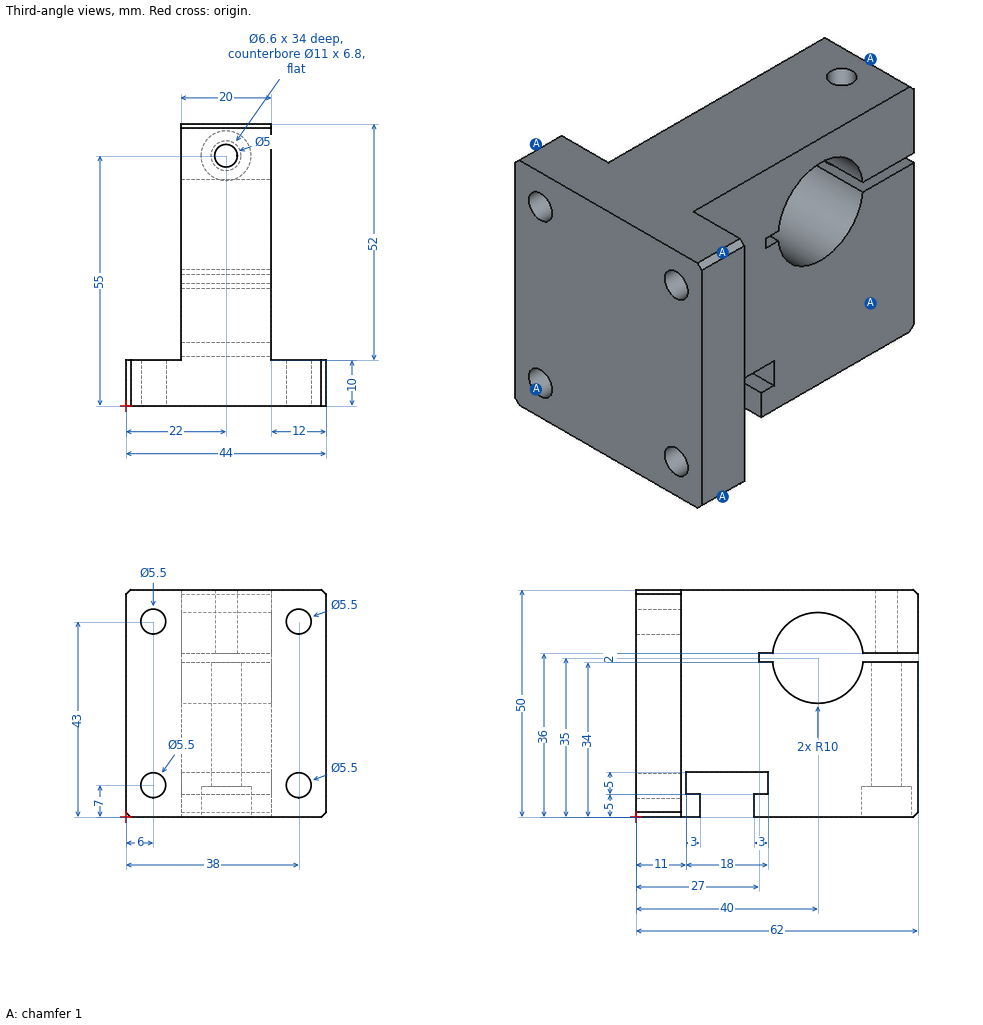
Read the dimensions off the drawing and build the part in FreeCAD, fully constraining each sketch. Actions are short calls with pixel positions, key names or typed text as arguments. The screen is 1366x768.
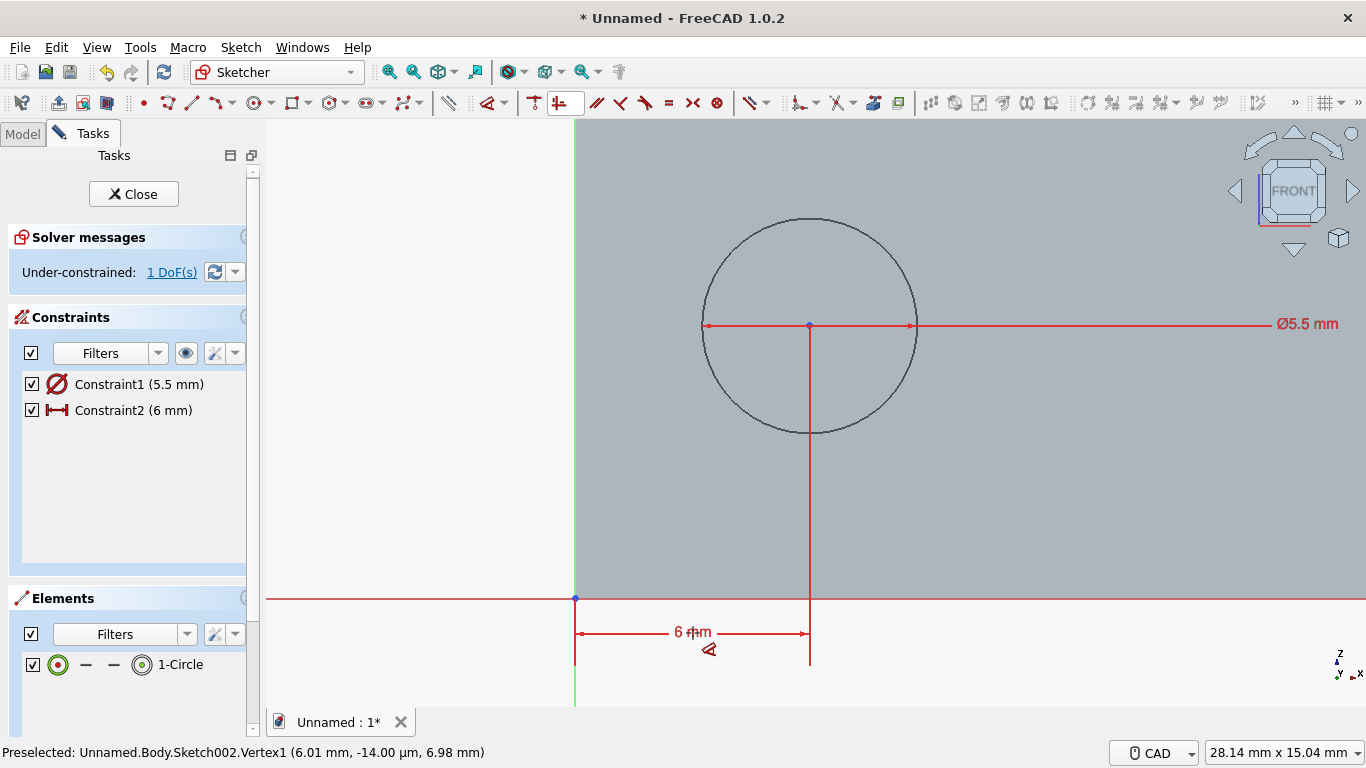
click(810, 326)
click(541, 462)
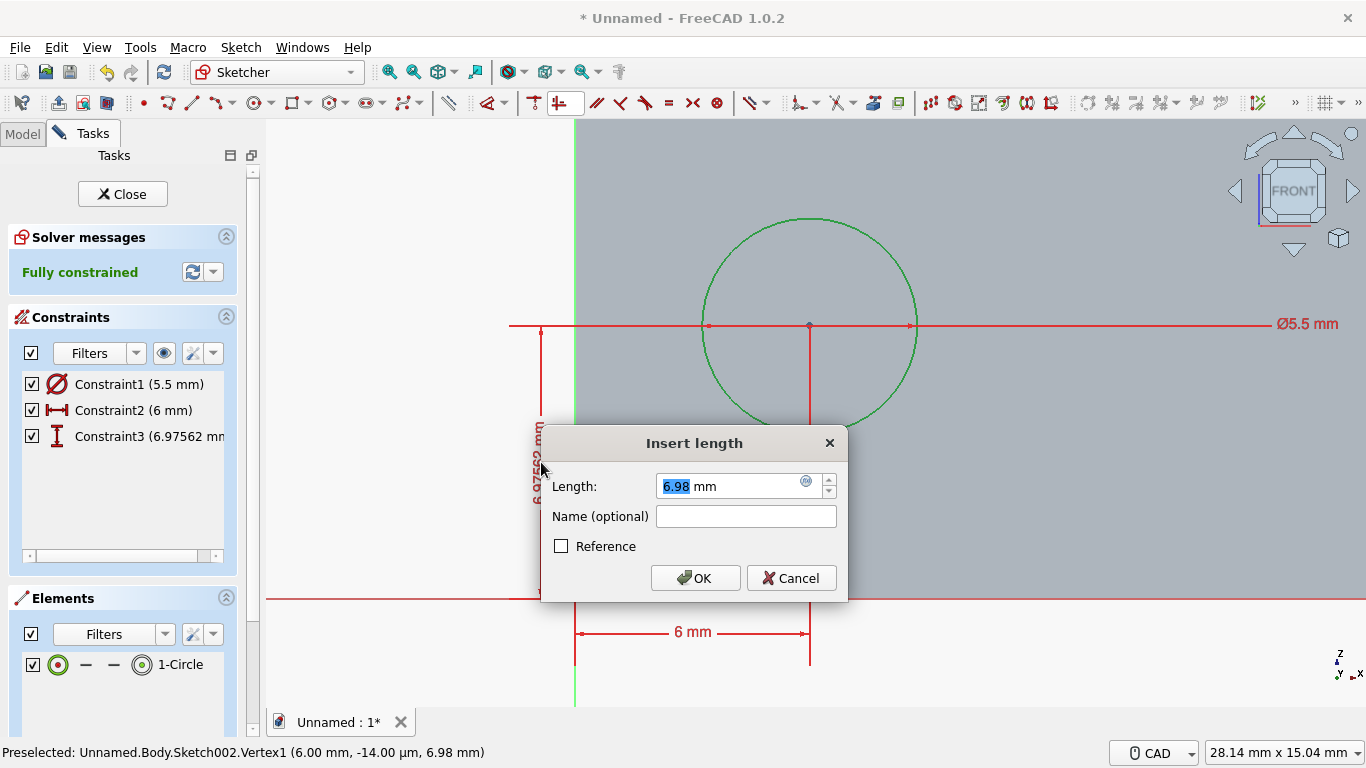
text(7)
key(Return)
key(Escape)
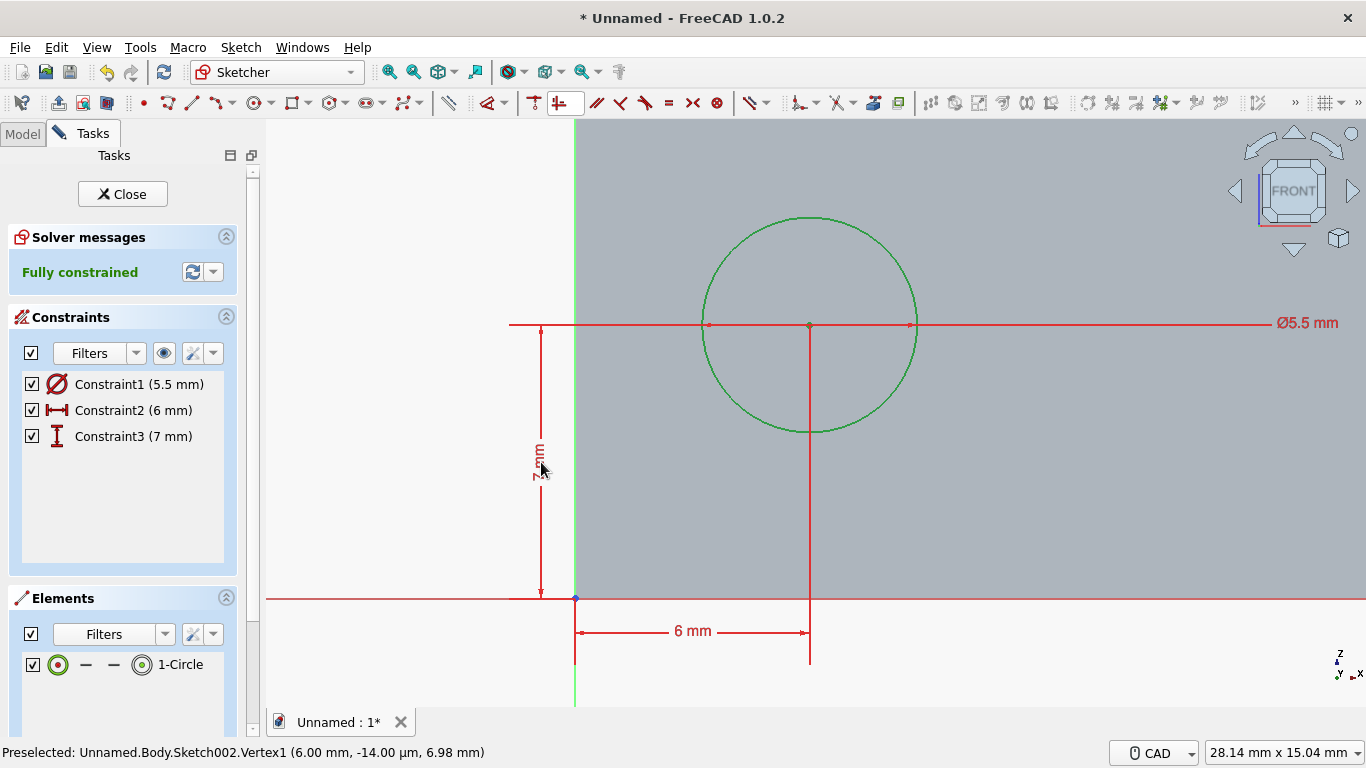
click(123, 194)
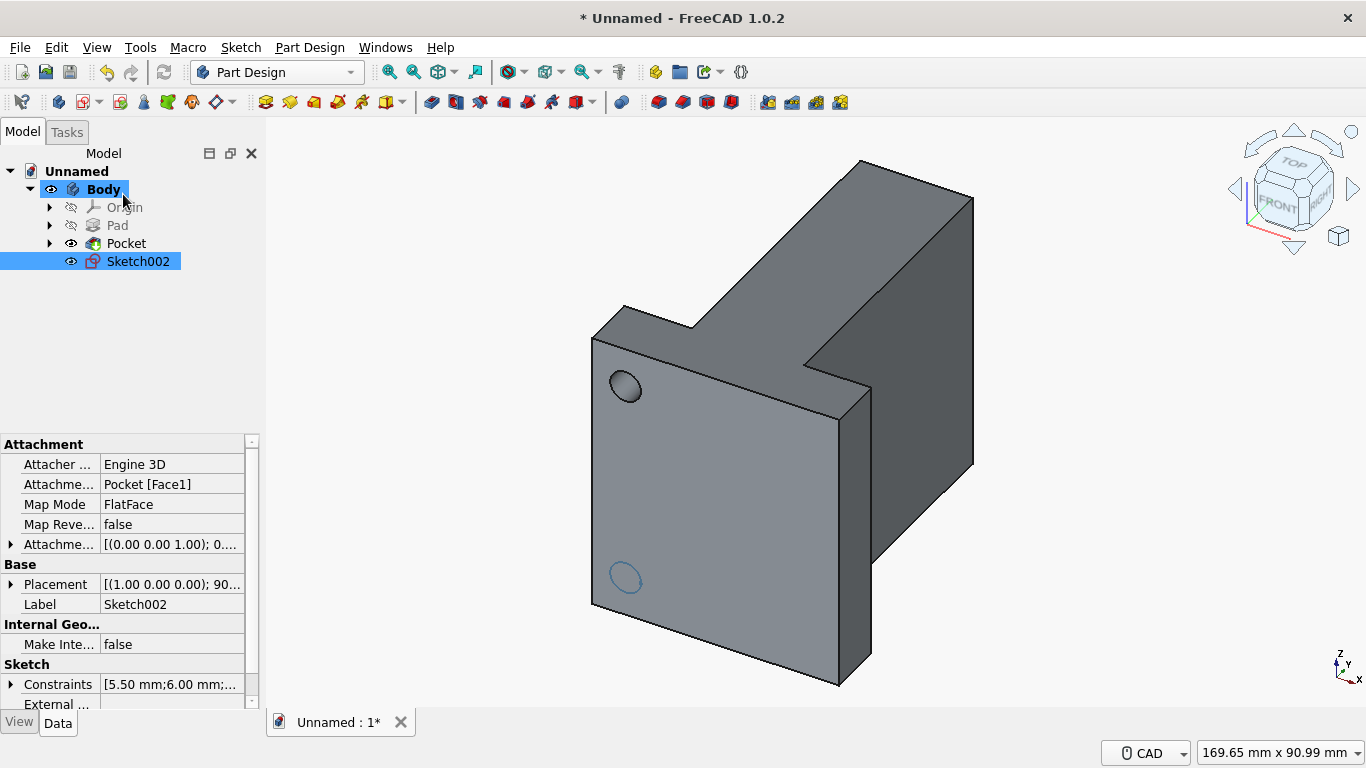
click(432, 102)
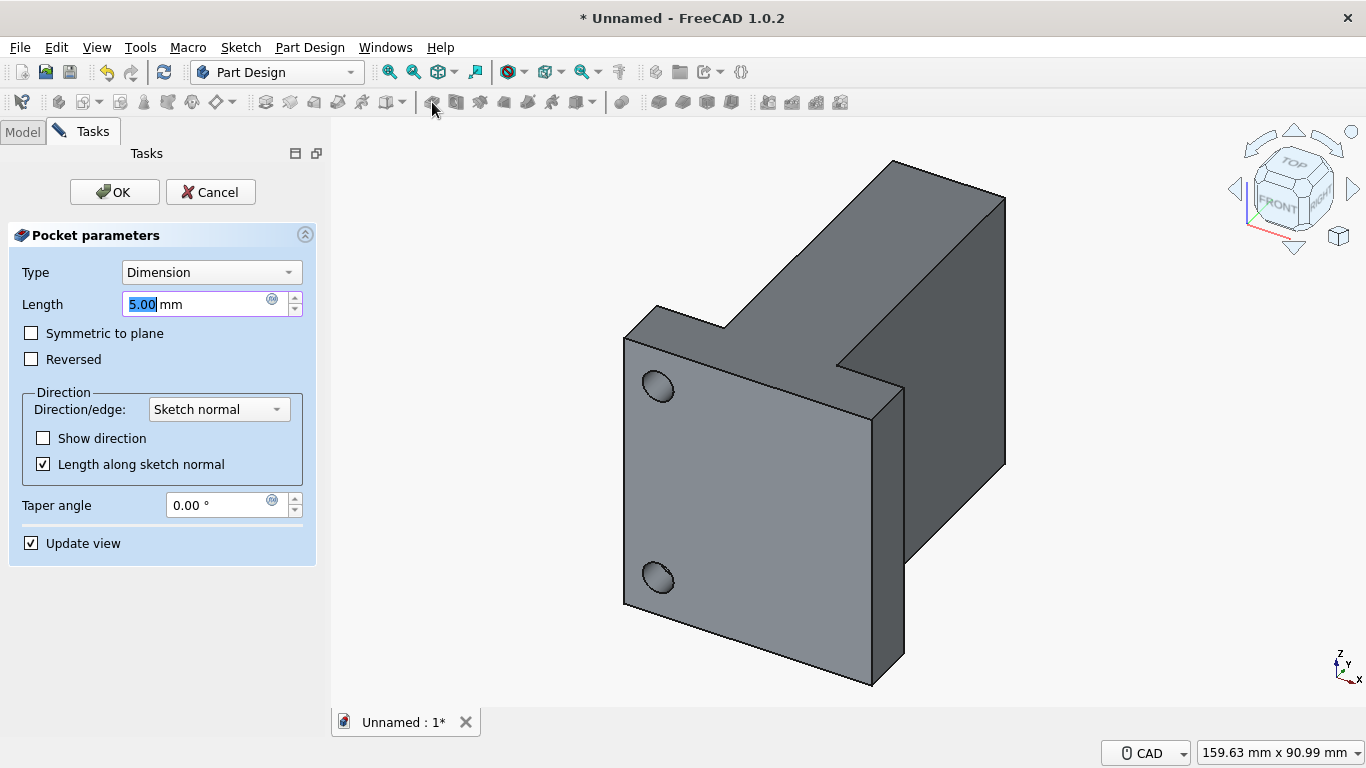
click(212, 272)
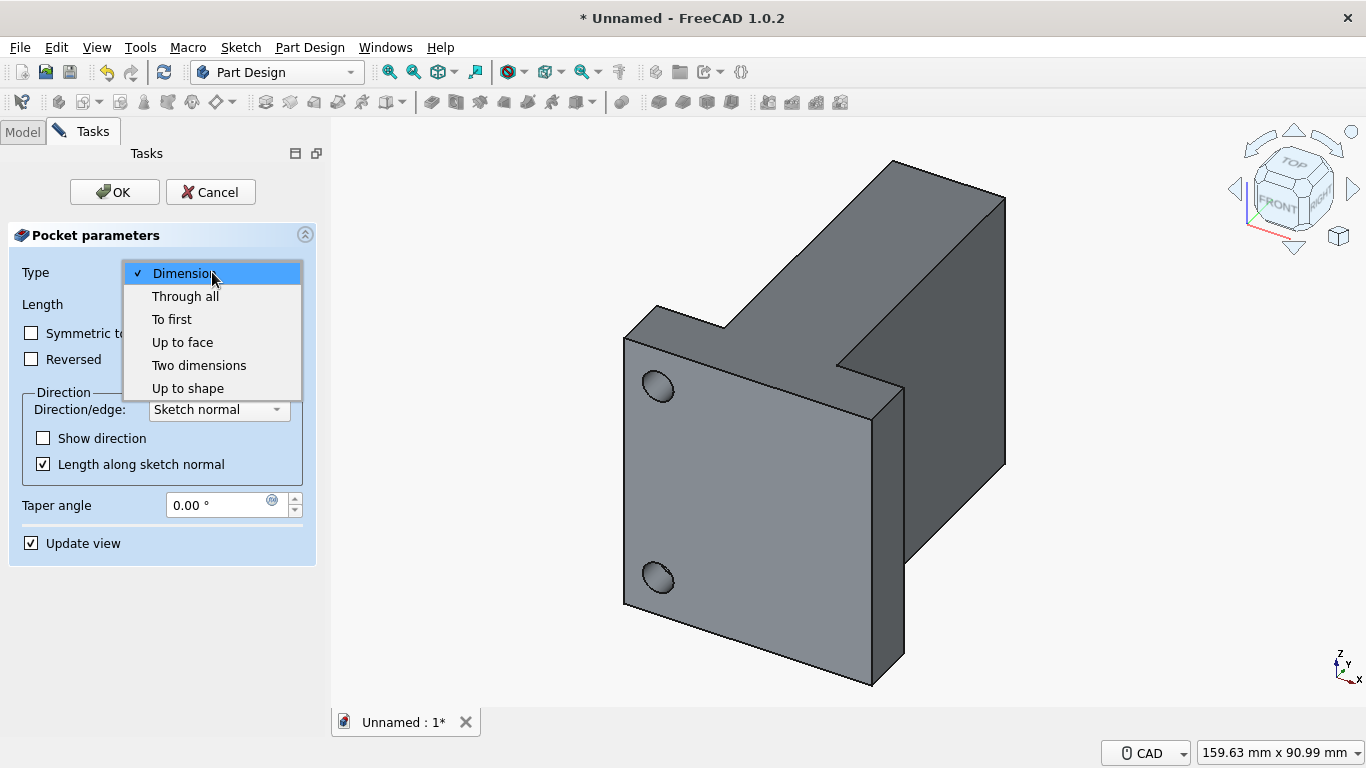
click(212, 320)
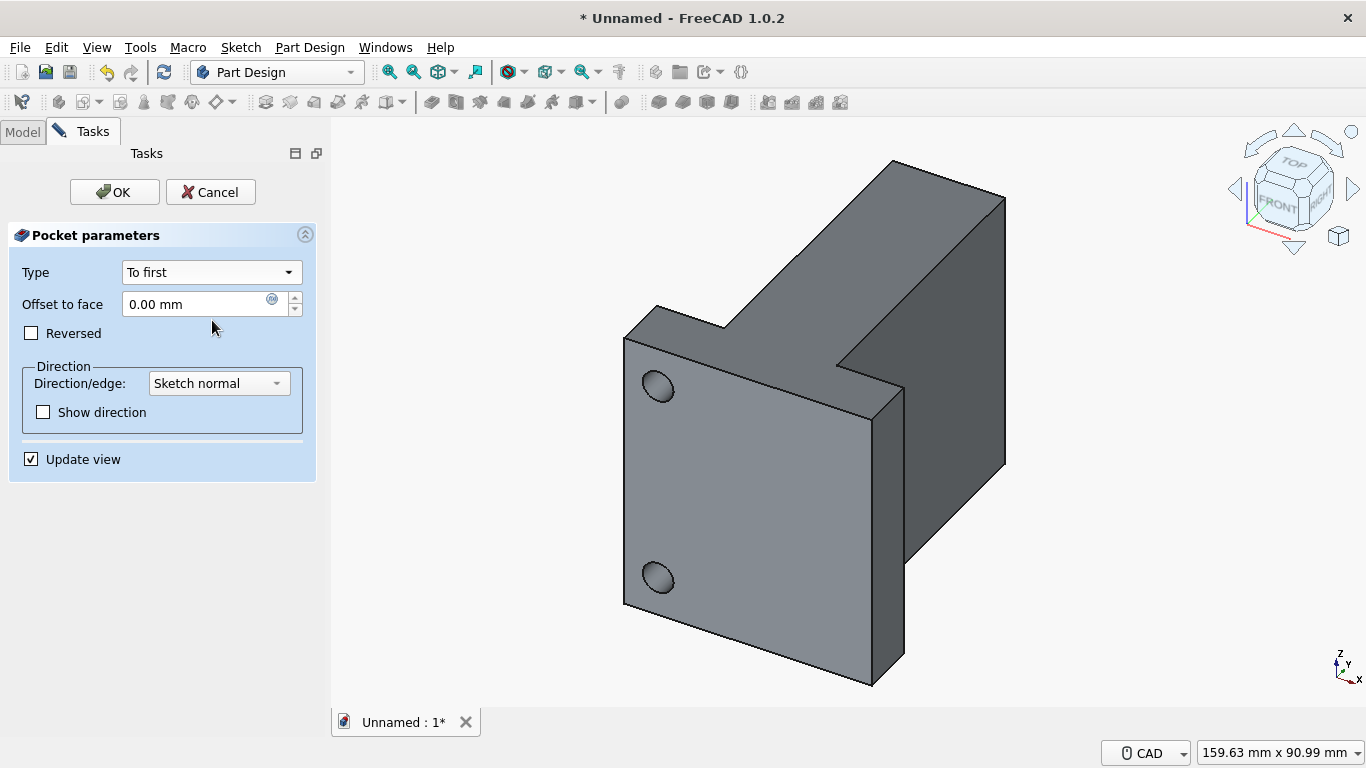
click(115, 192)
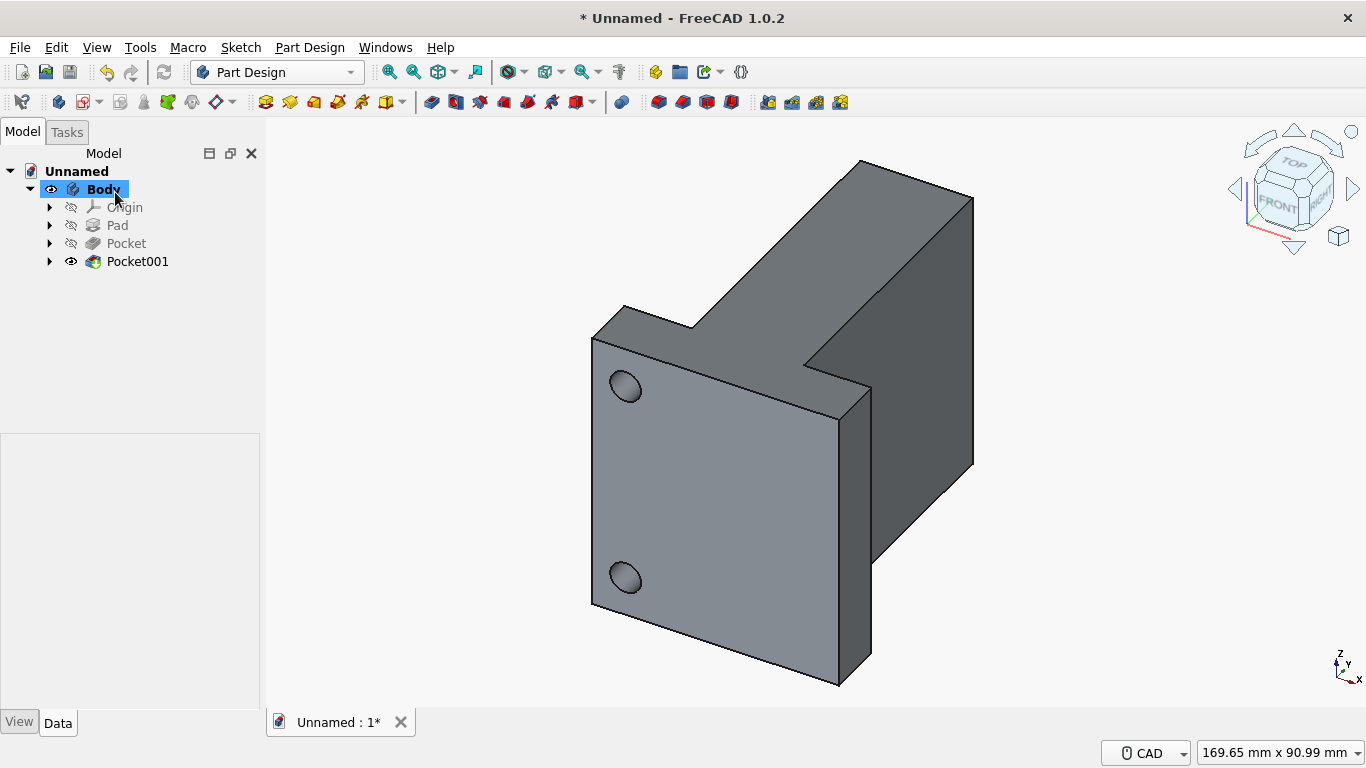
click(715, 511)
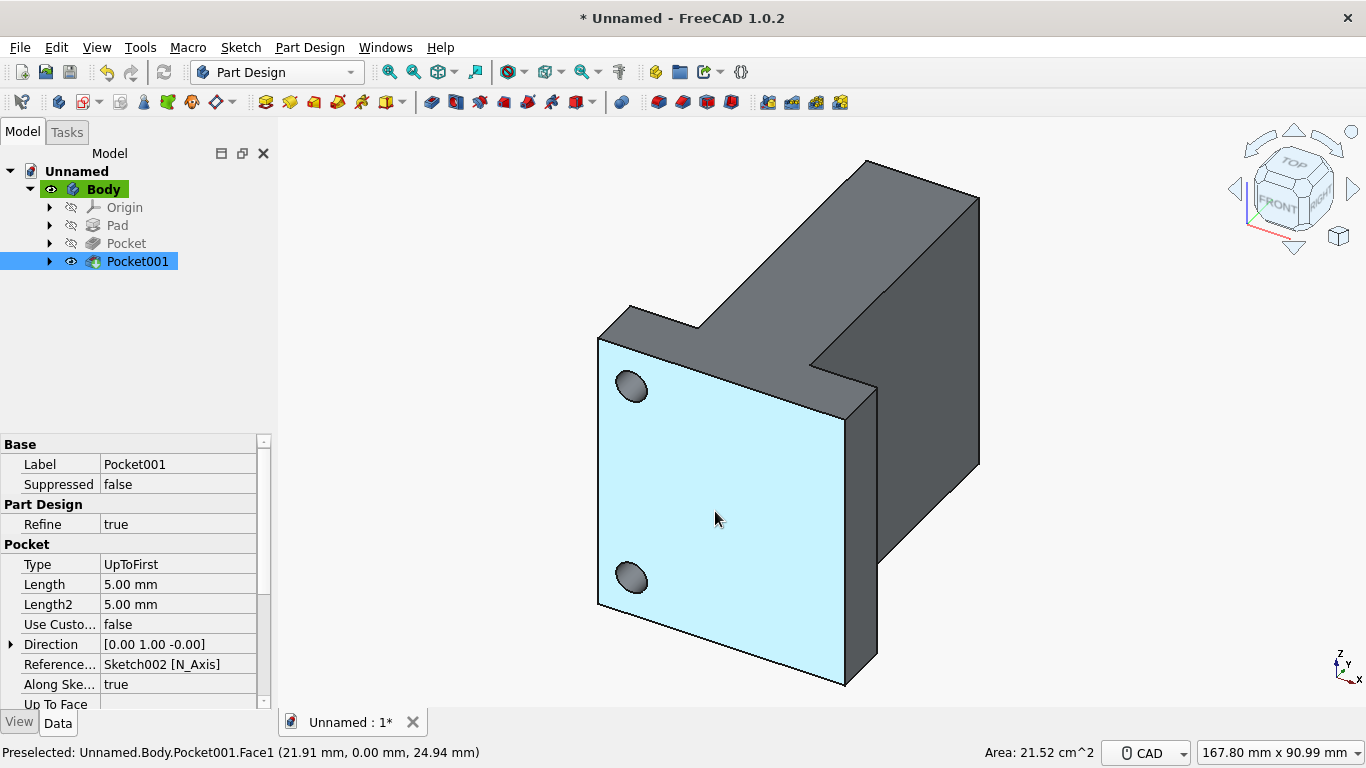
click(84, 102)